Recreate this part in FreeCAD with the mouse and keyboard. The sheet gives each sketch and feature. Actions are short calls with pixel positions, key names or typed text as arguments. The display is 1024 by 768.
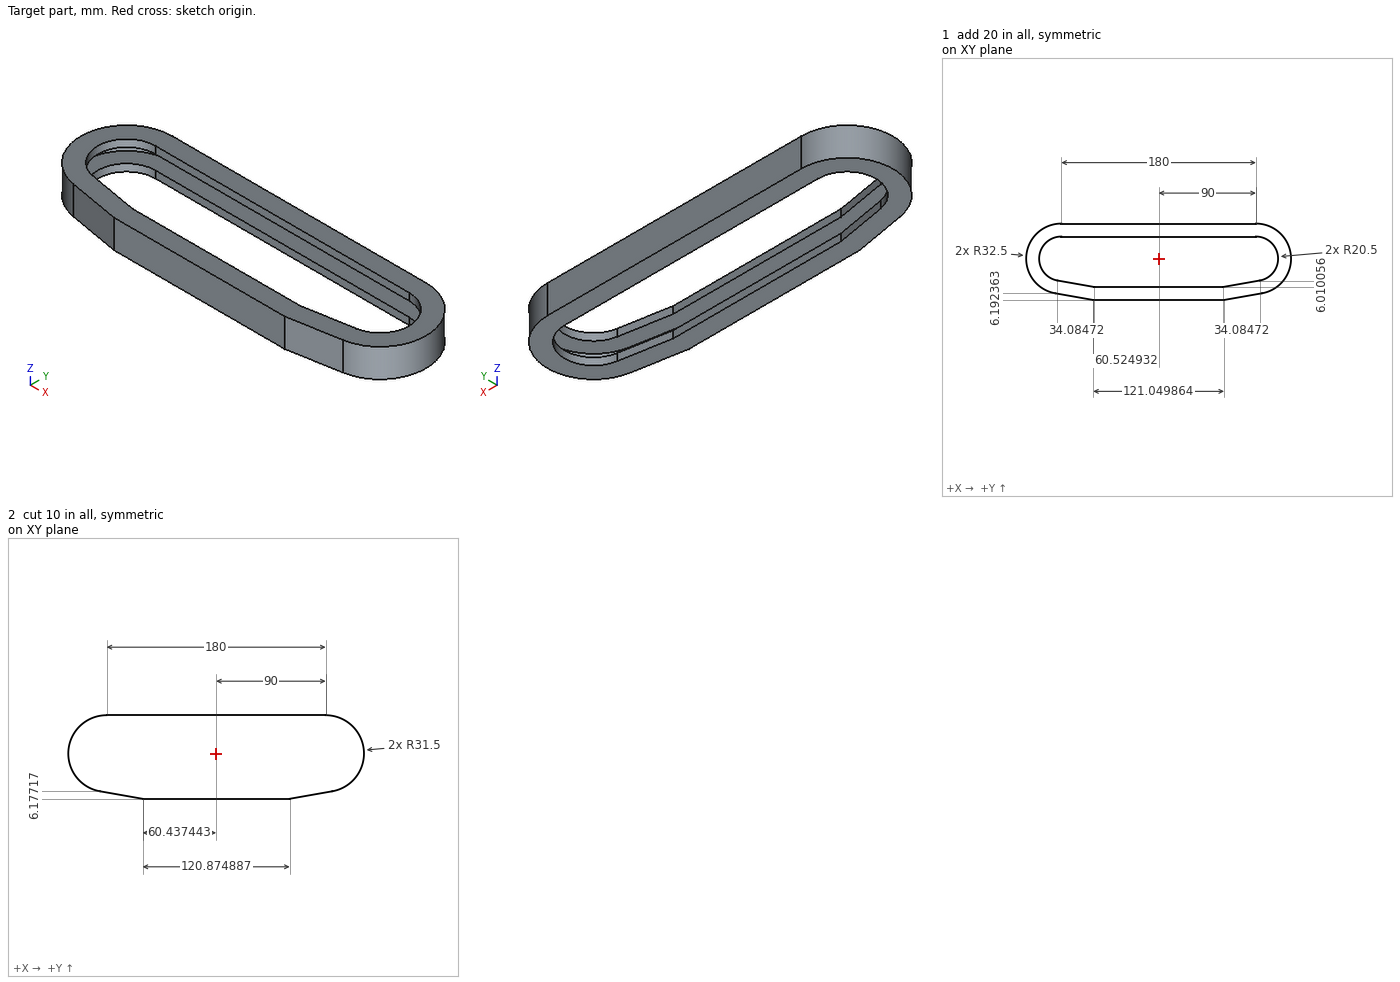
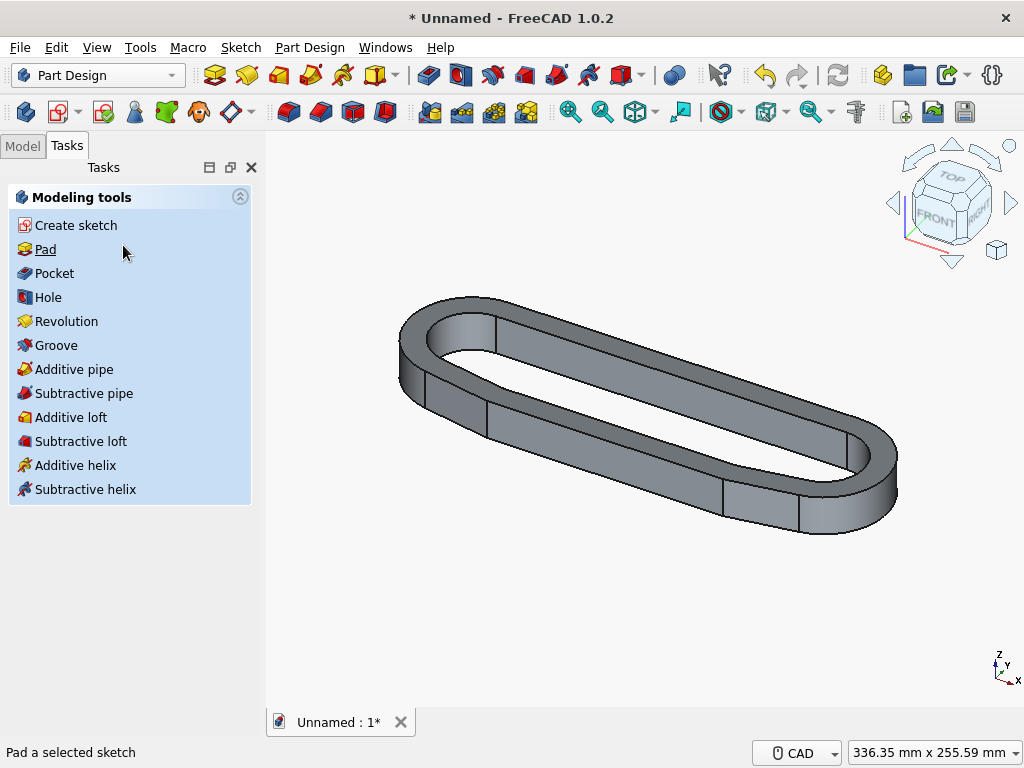
click(430, 76)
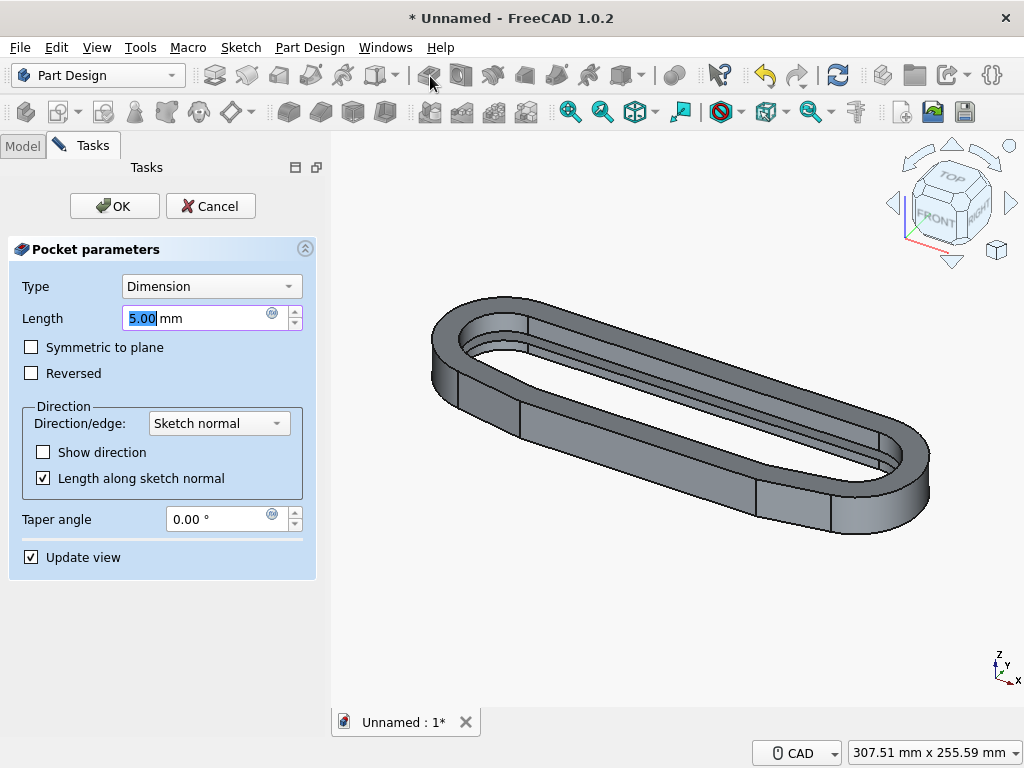
text(10)
key(Tab)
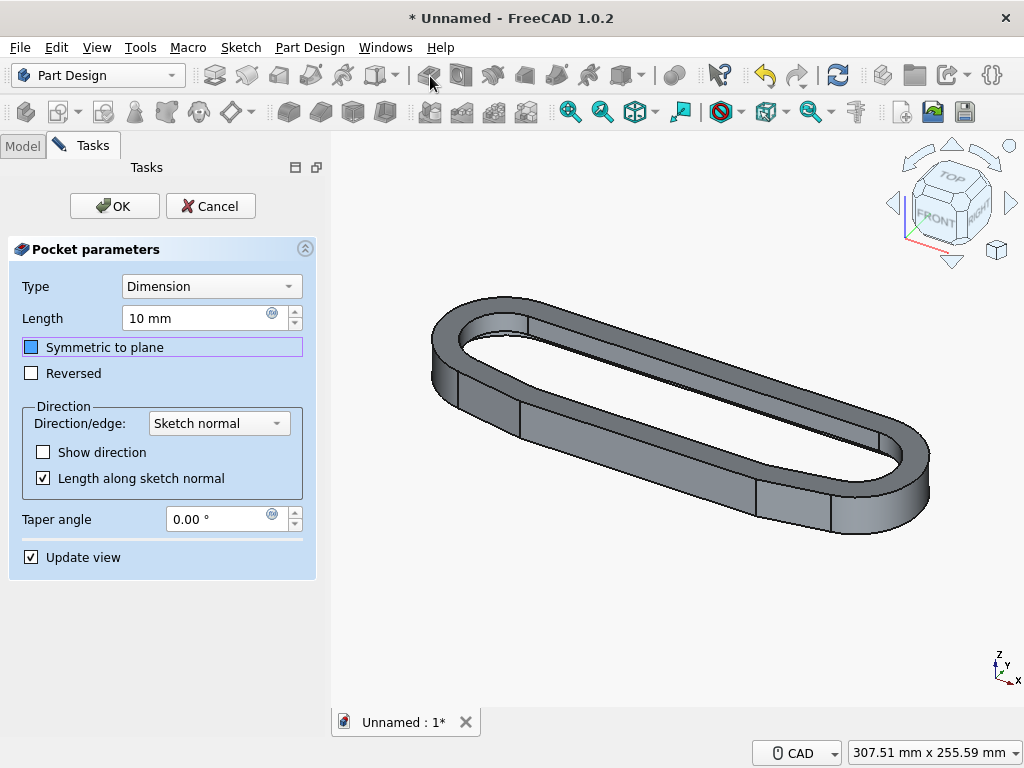
click(30, 347)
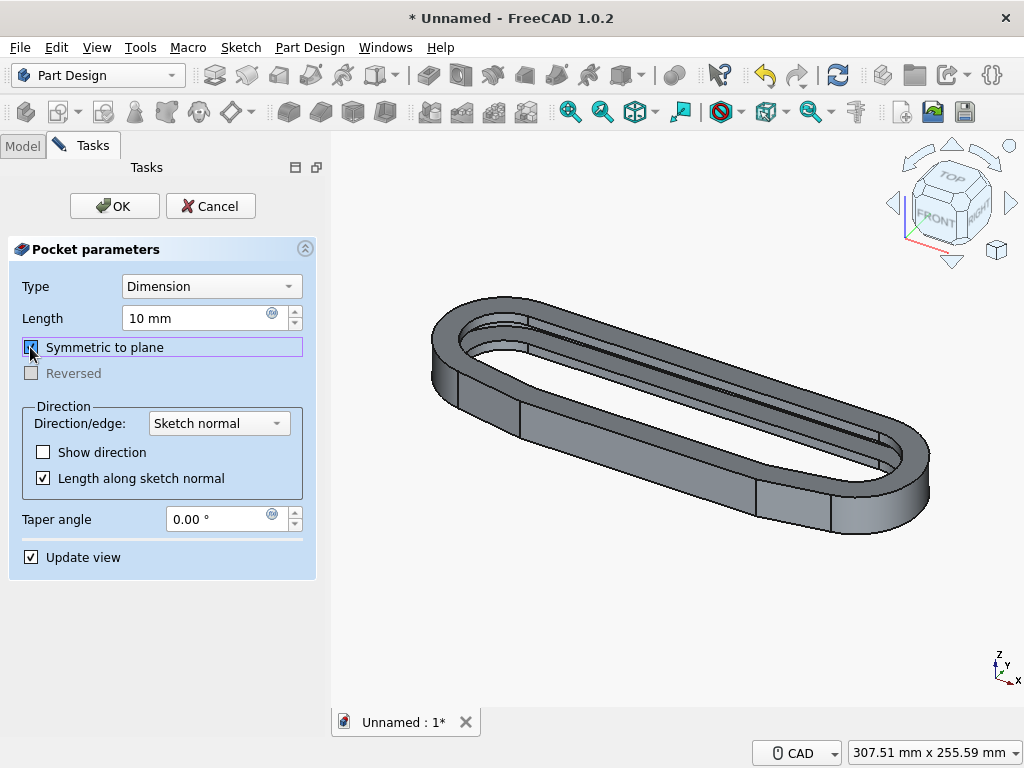
click(115, 206)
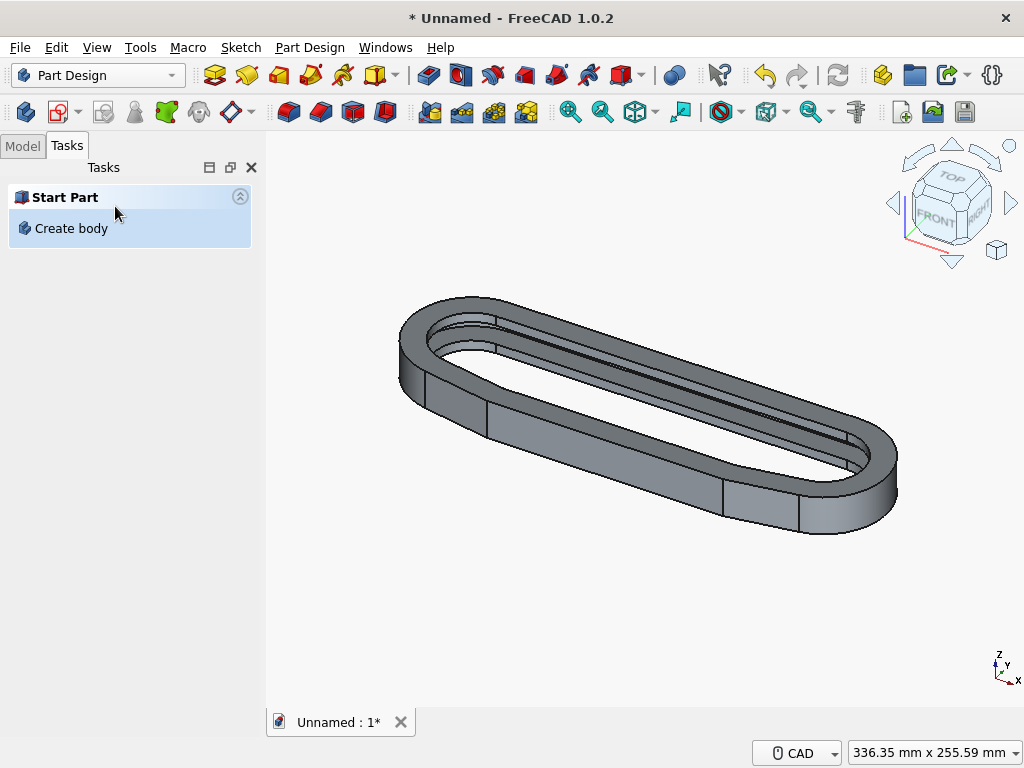
key(0)